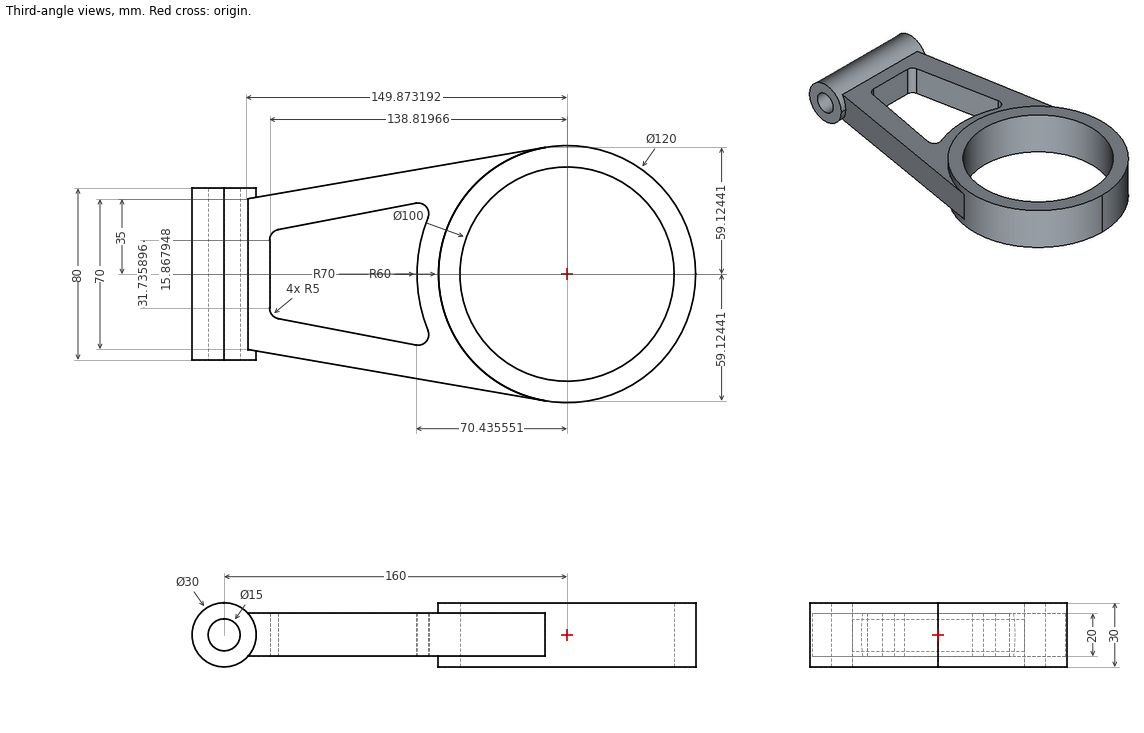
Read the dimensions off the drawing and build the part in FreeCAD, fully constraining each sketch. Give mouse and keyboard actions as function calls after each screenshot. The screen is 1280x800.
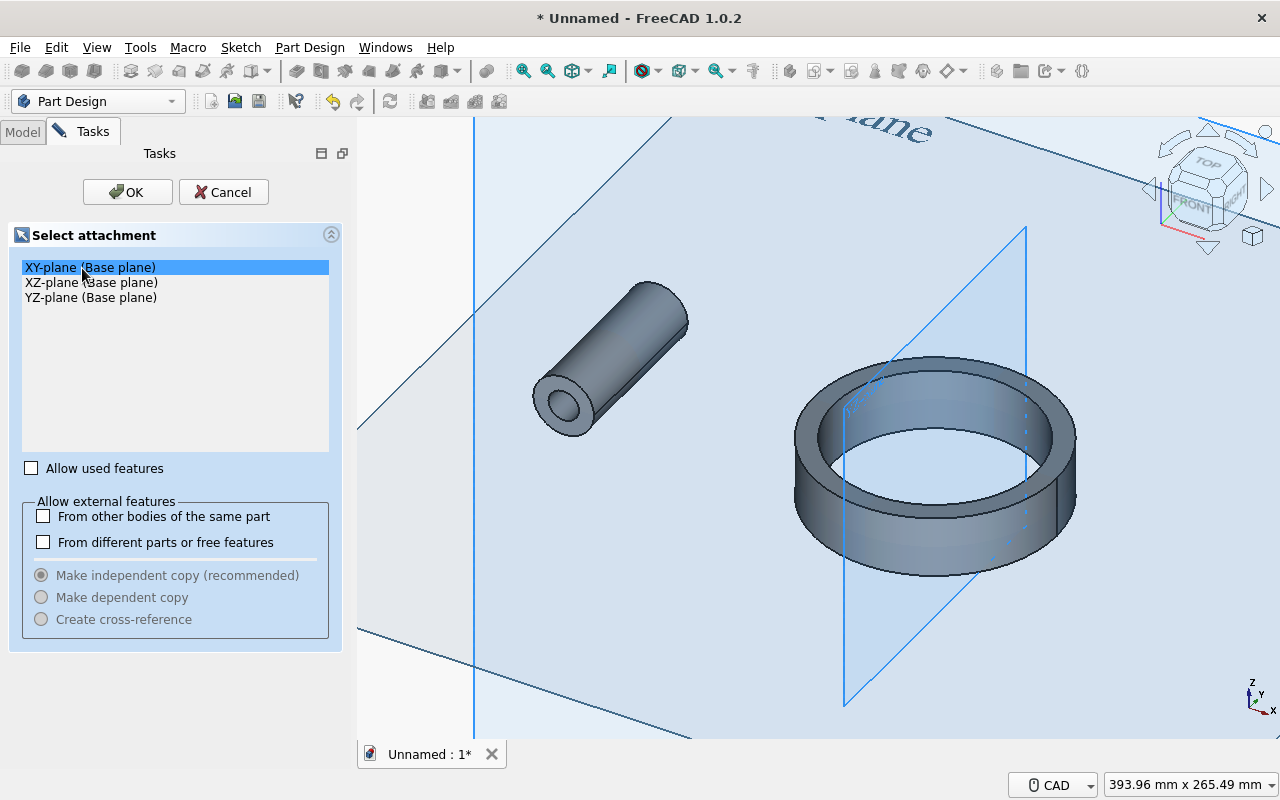
click(128, 192)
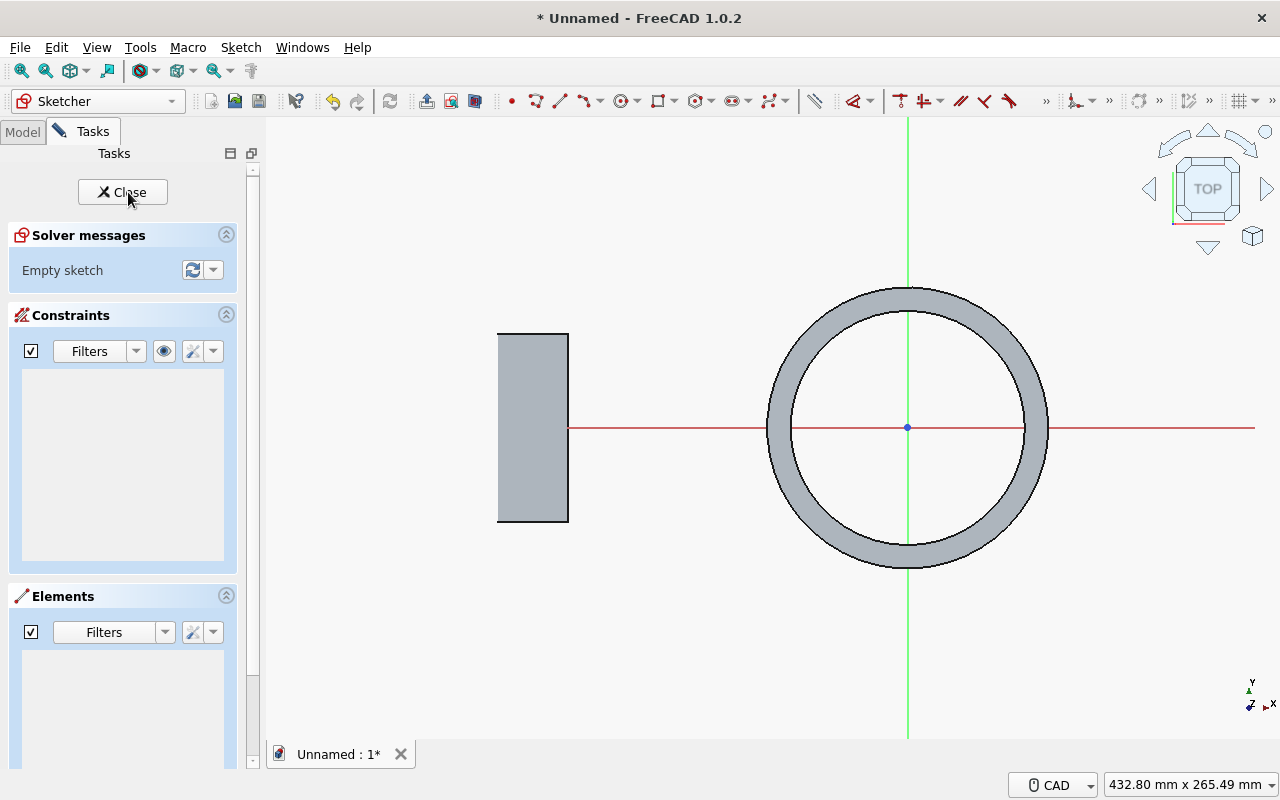
click(476, 102)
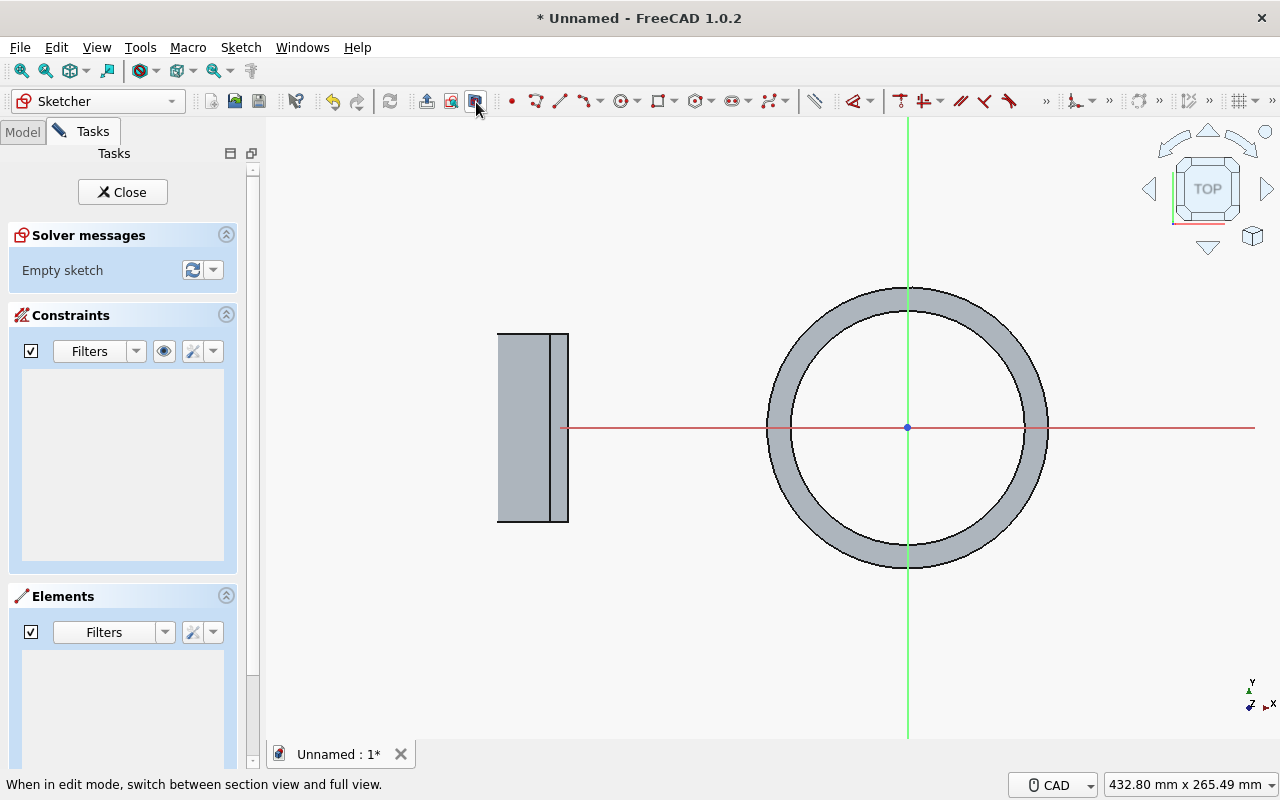
scroll(788, 428, up, 2)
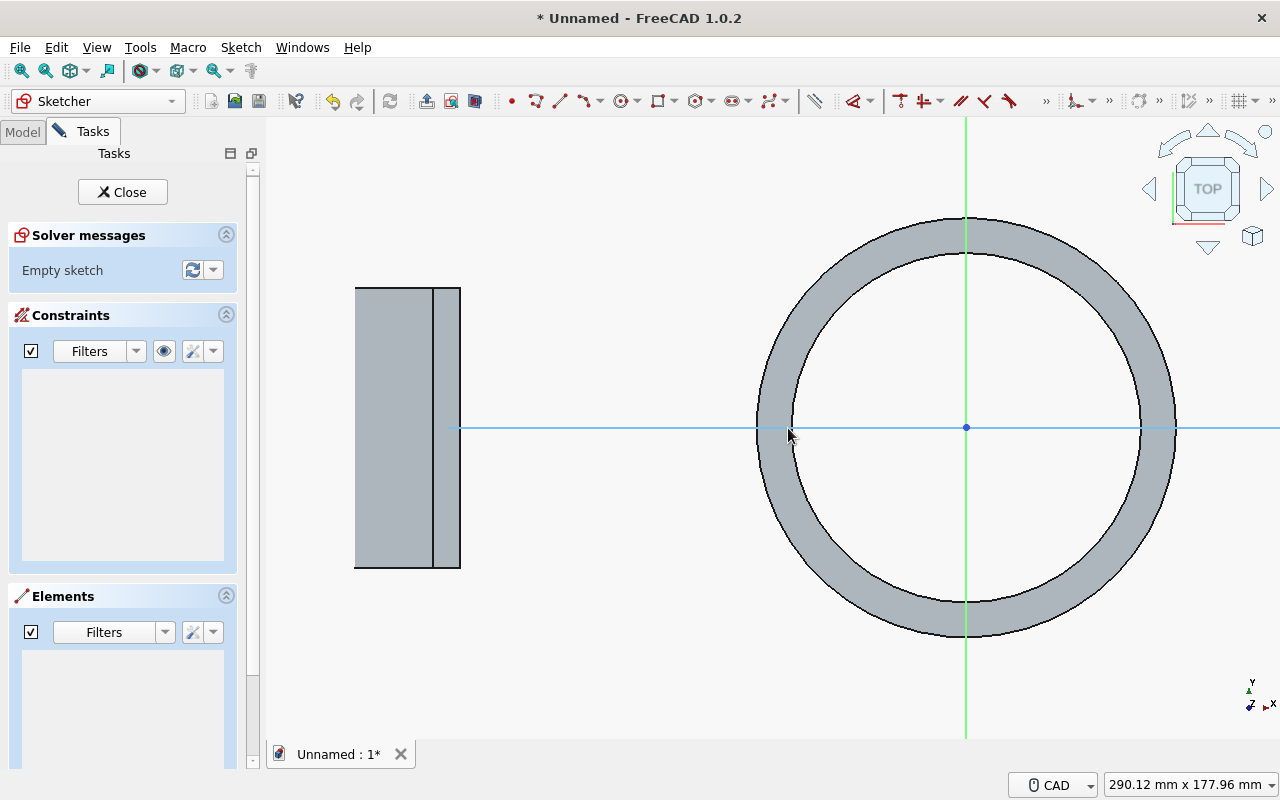
click(536, 102)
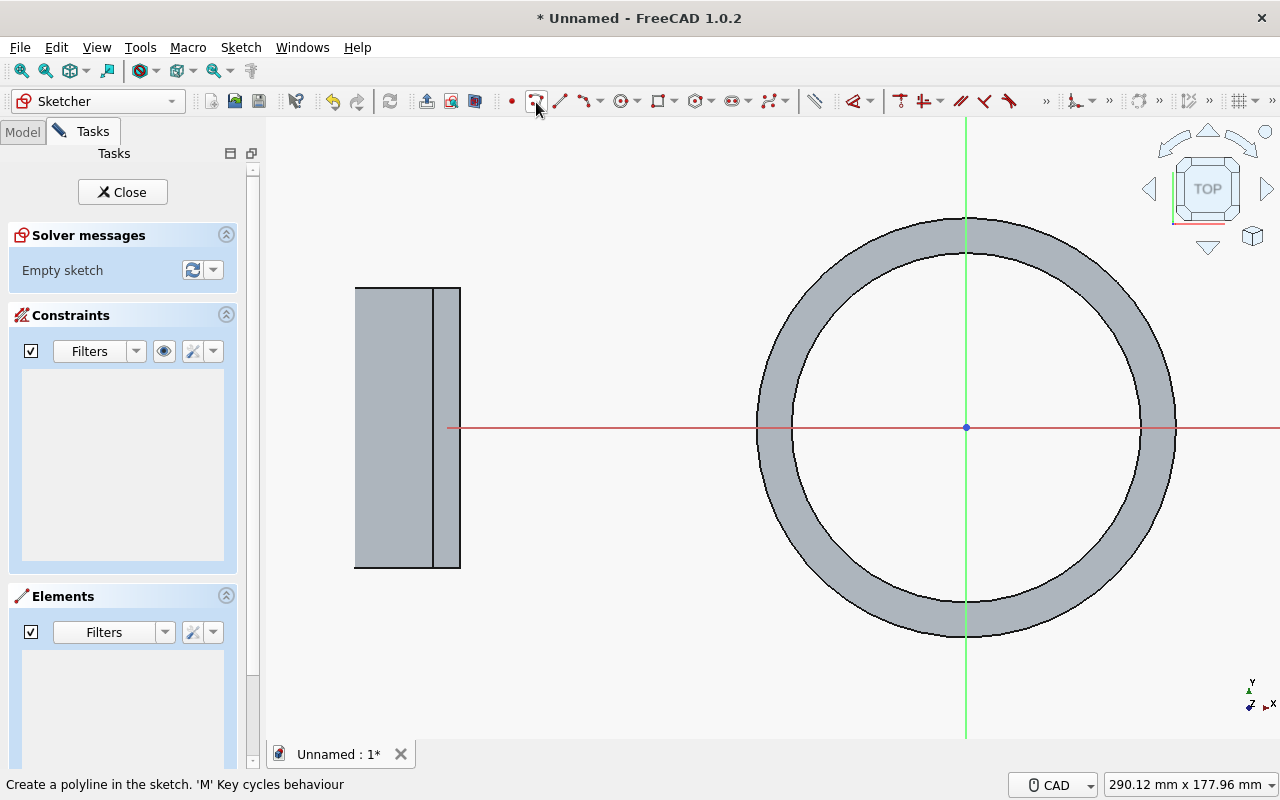
click(931, 221)
click(443, 305)
click(443, 550)
click(931, 634)
right_click(931, 634)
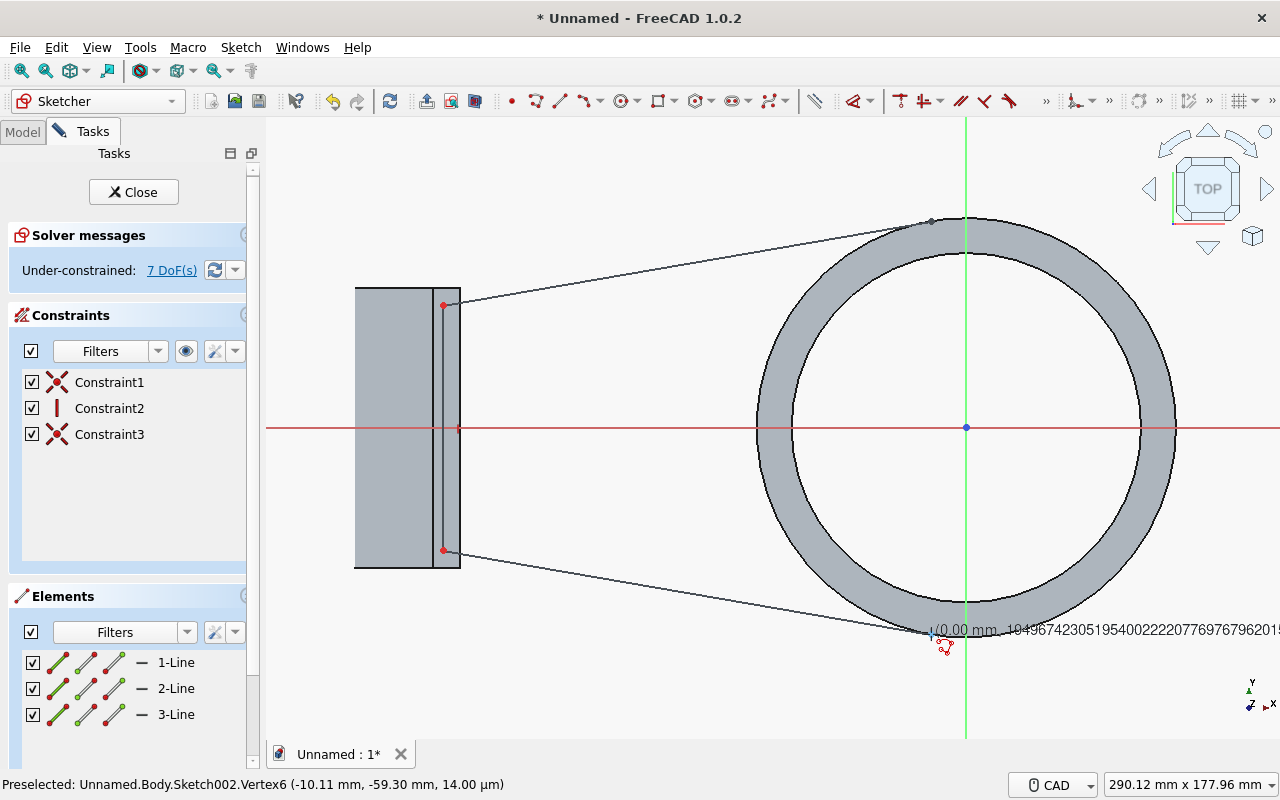
click(584, 102)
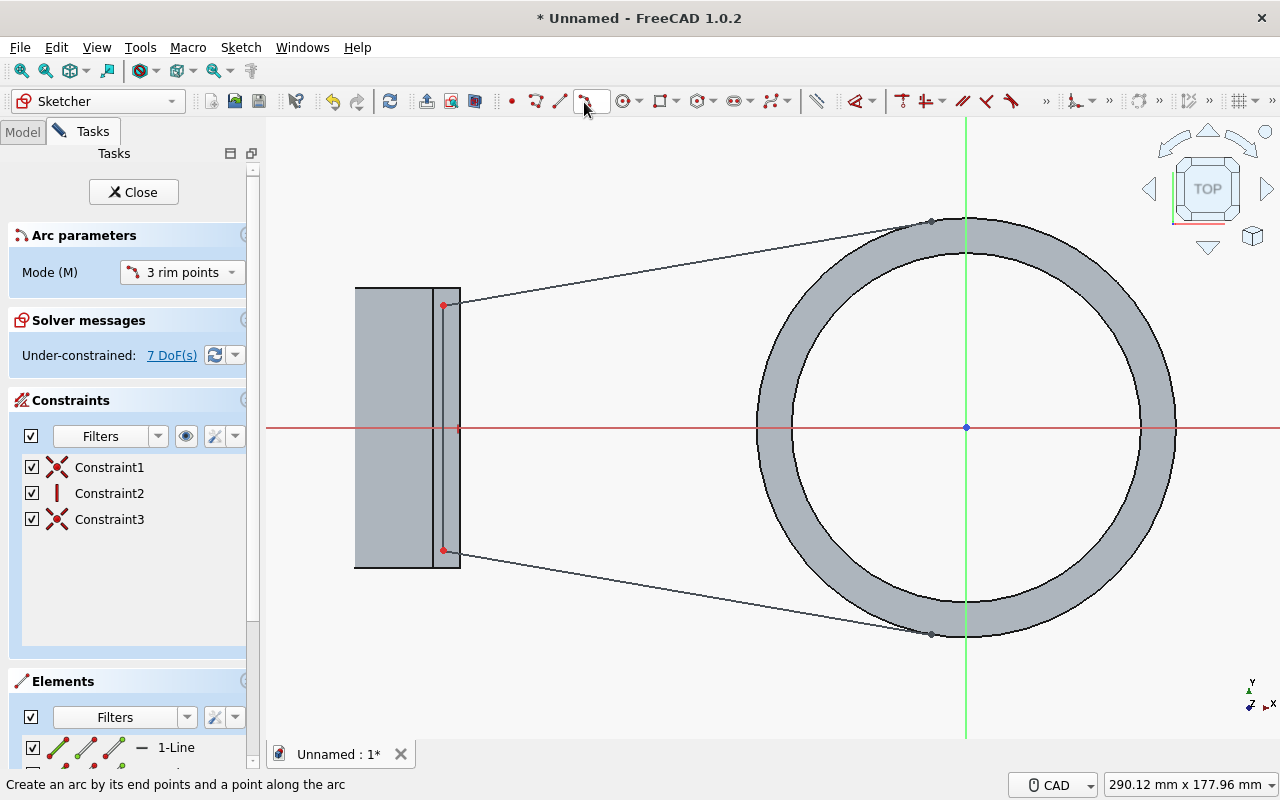
click(931, 635)
click(931, 222)
click(765, 370)
key(Escape)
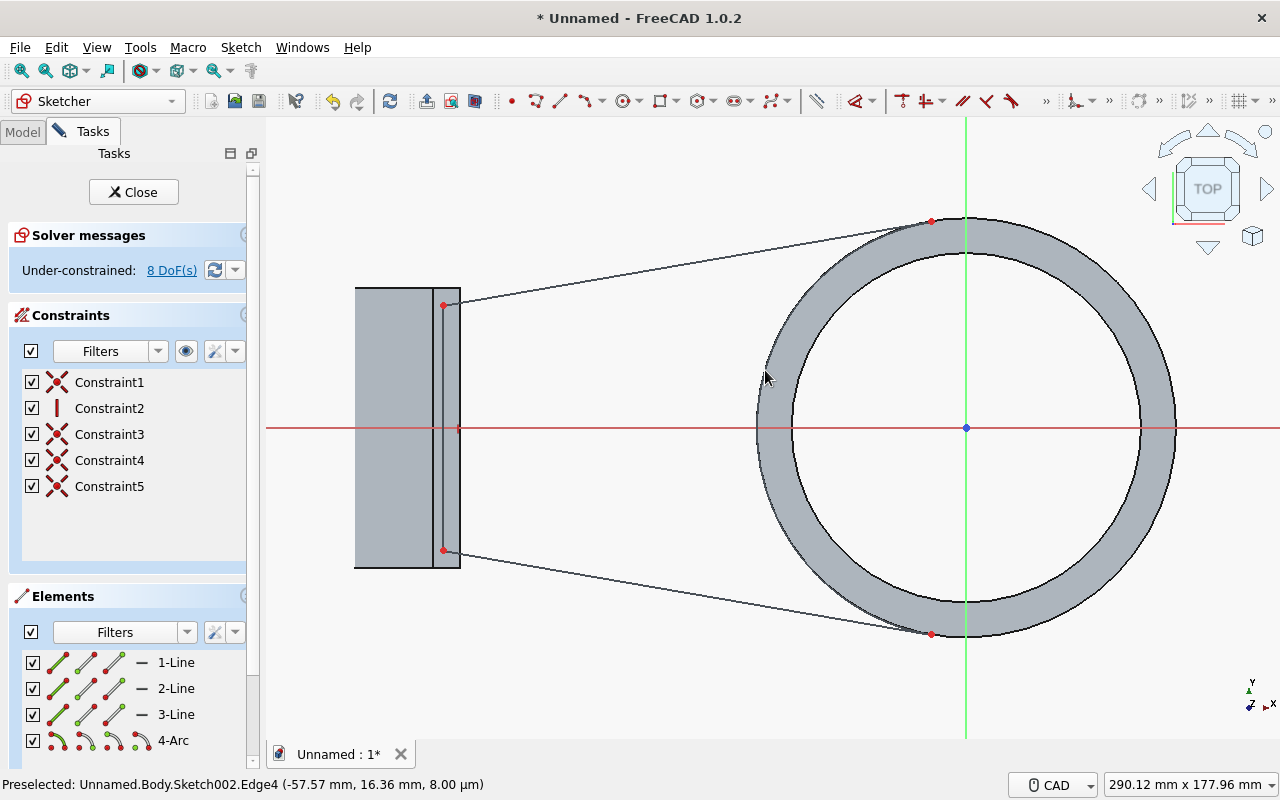
drag(956, 418, 976, 439)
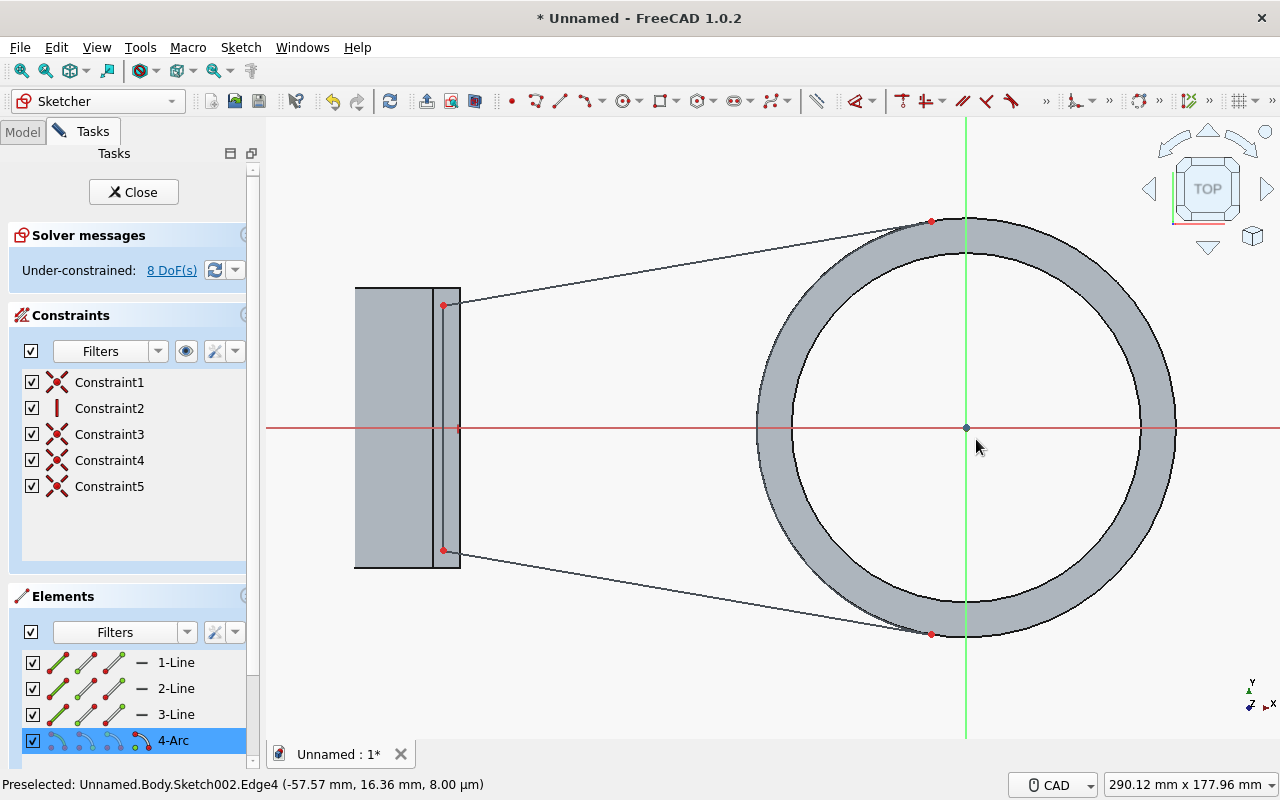
click(902, 102)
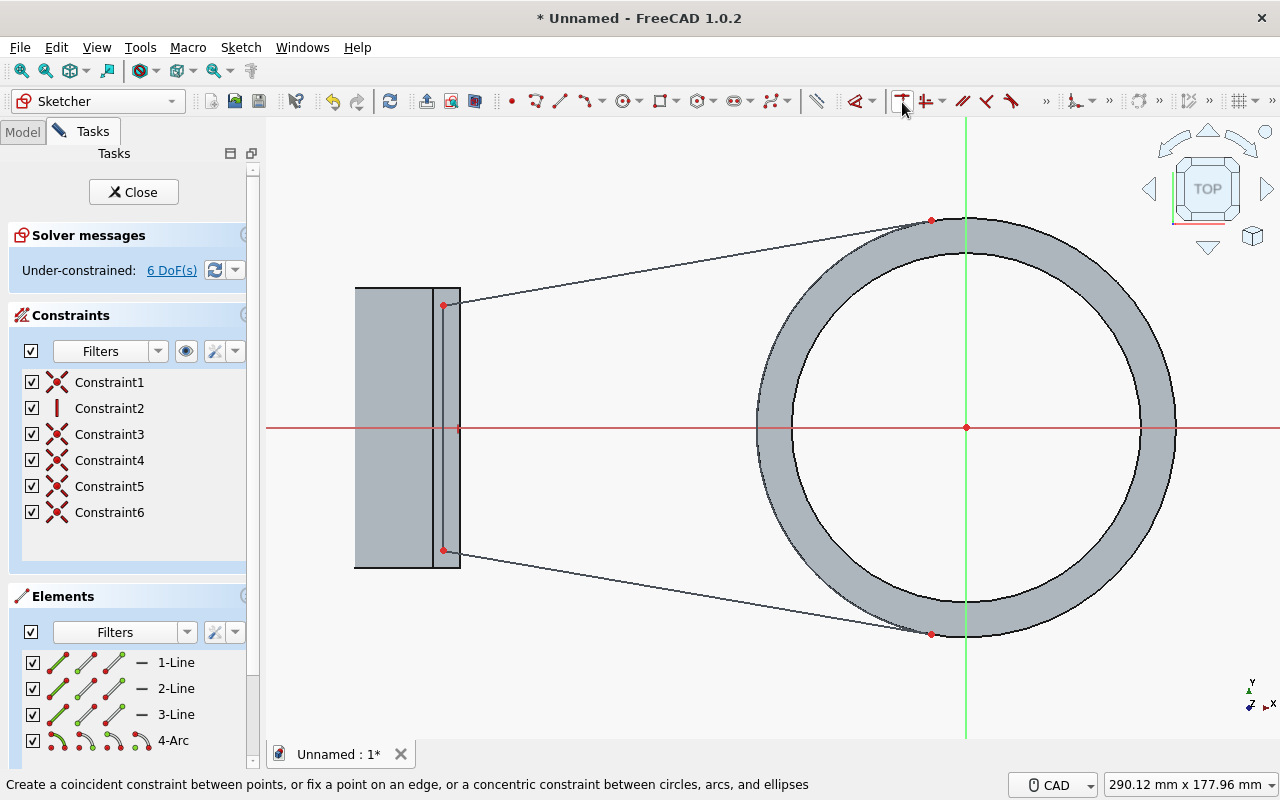
click(856, 102)